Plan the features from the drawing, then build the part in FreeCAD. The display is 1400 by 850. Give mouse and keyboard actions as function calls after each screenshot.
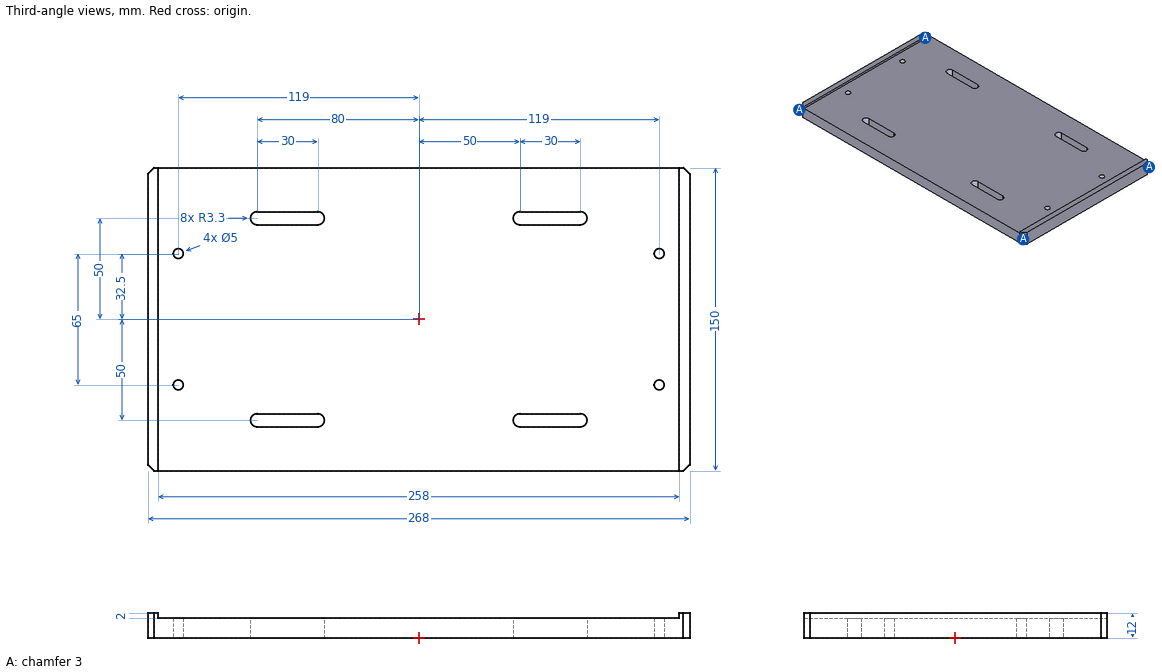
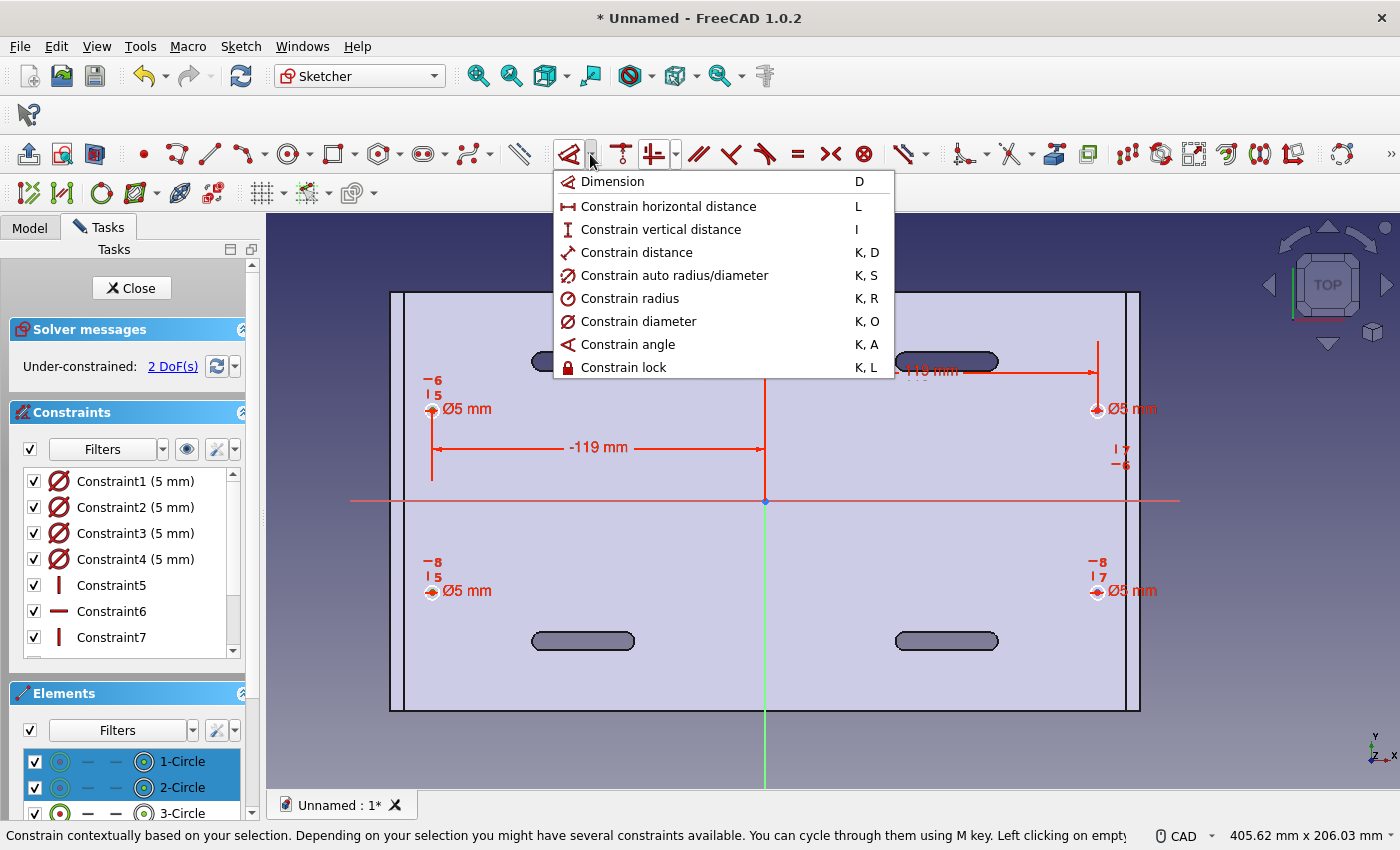
click(724, 230)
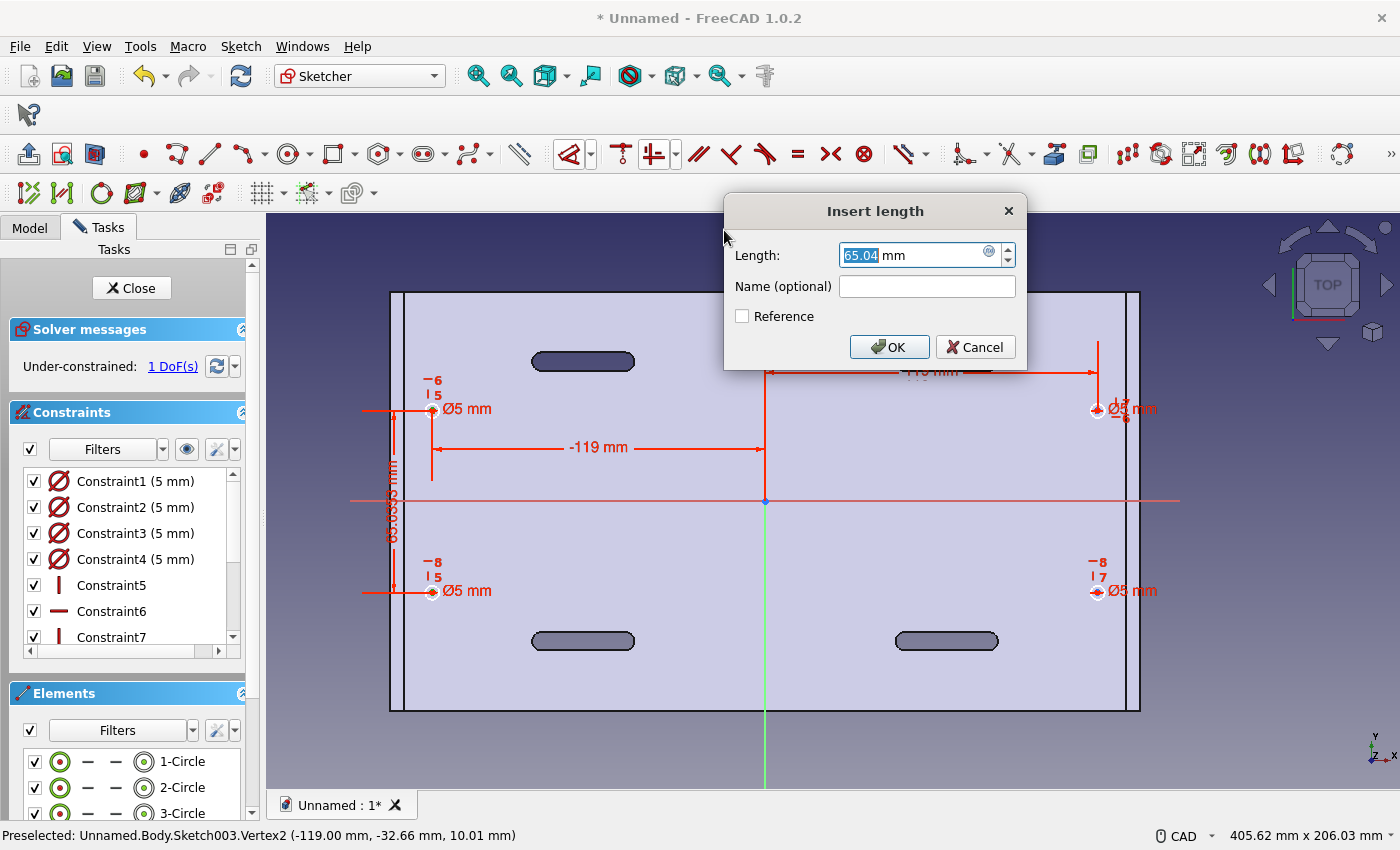
text(65)
key(Return)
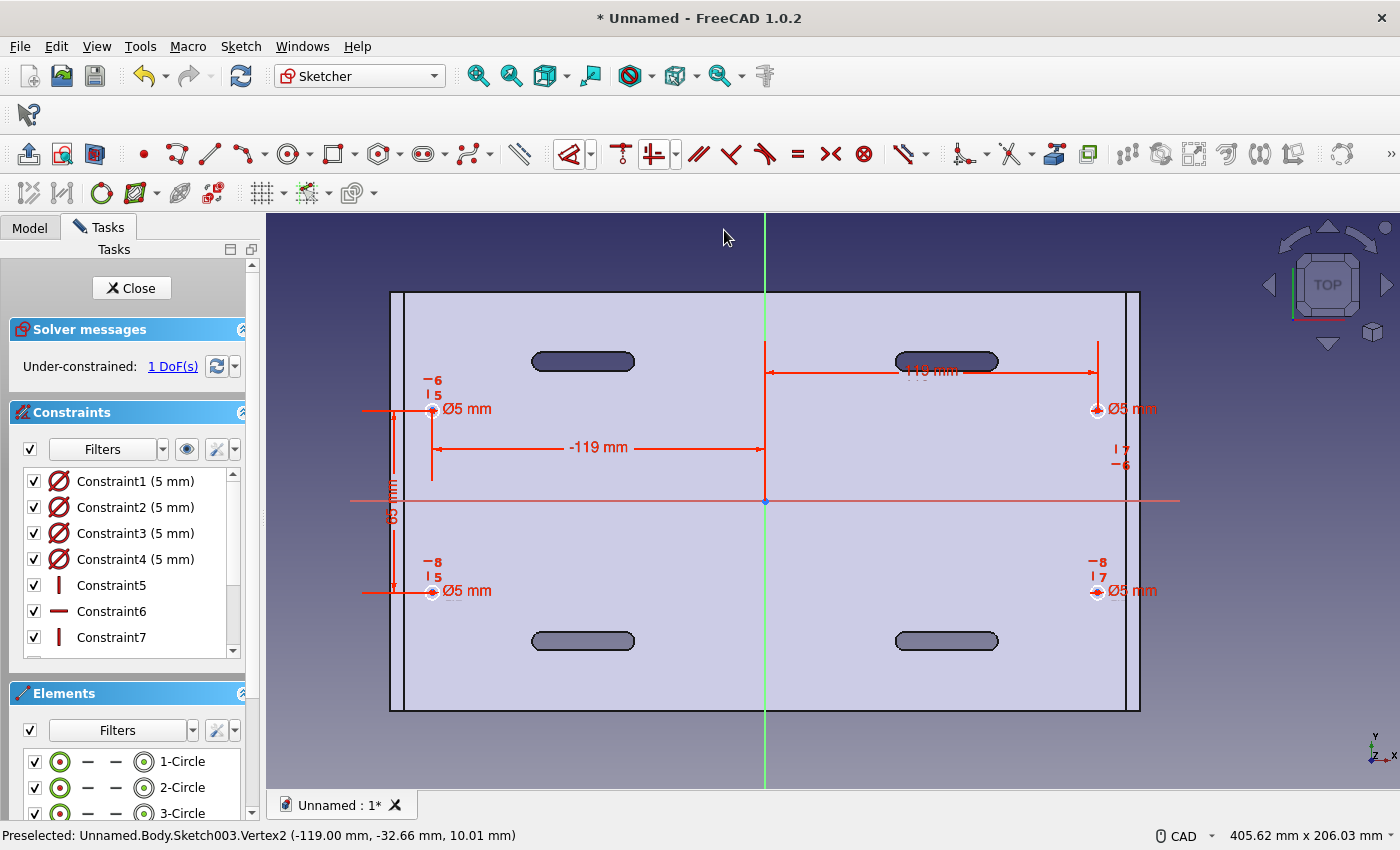
click(432, 411)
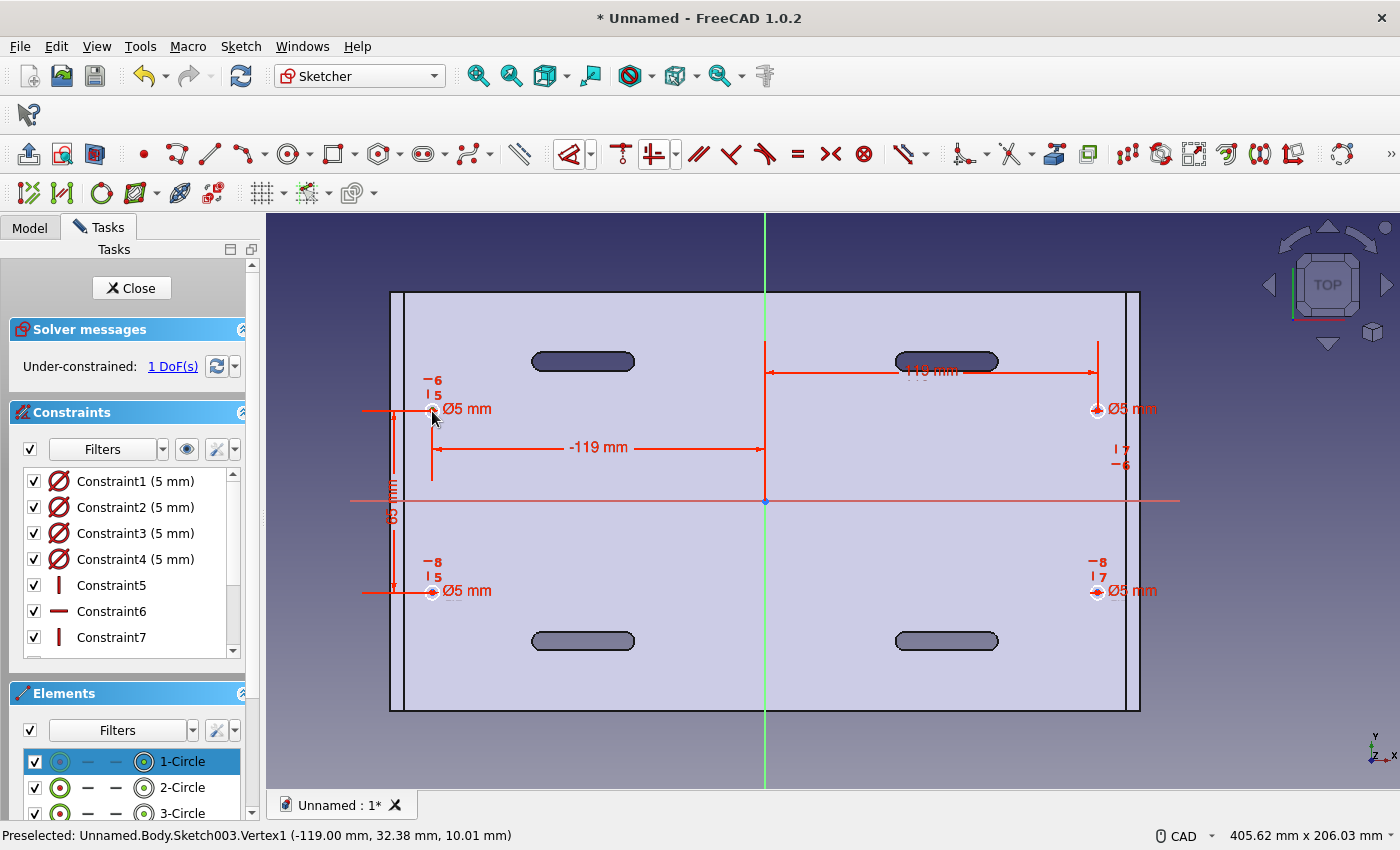
click(590, 154)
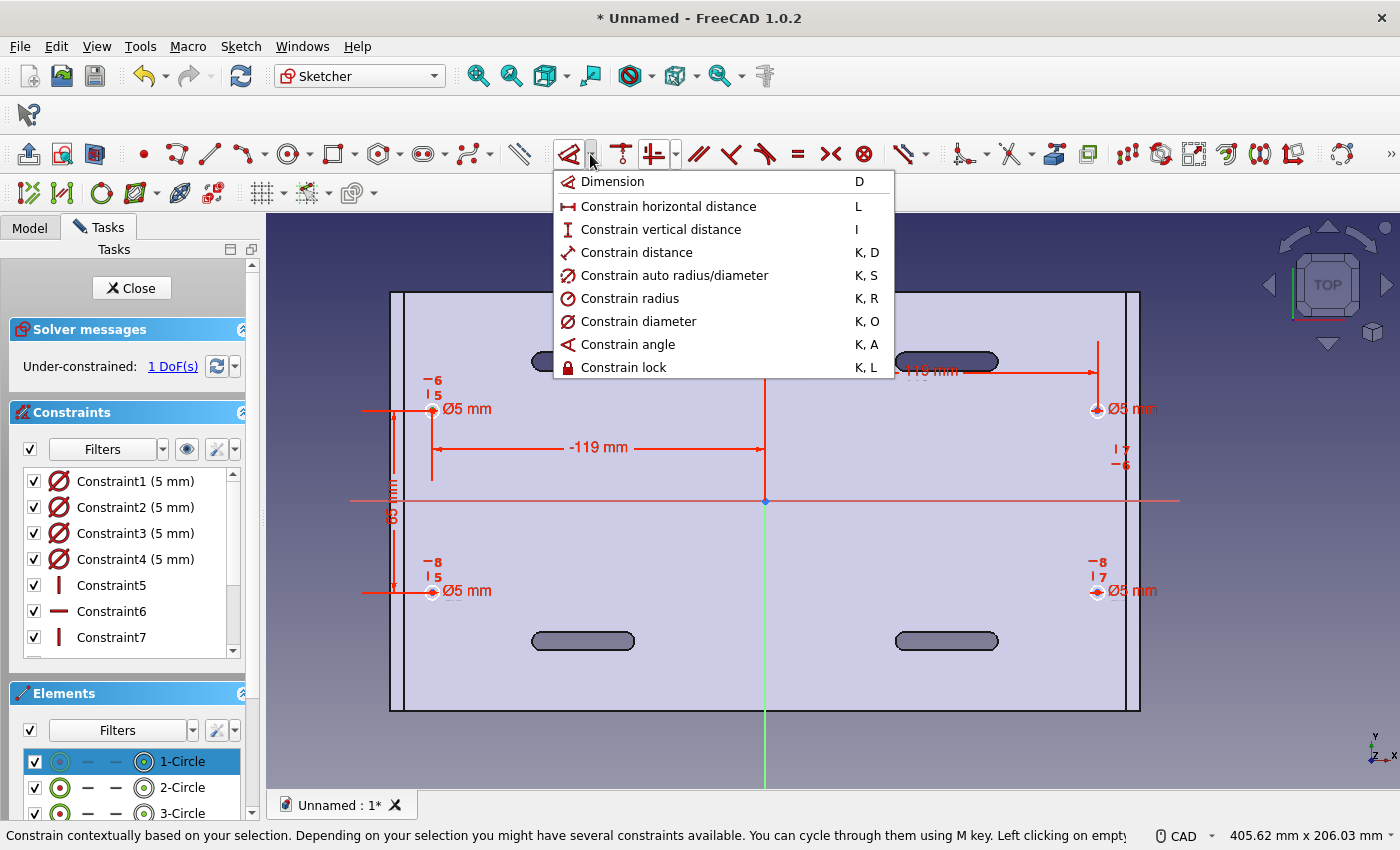
click(724, 230)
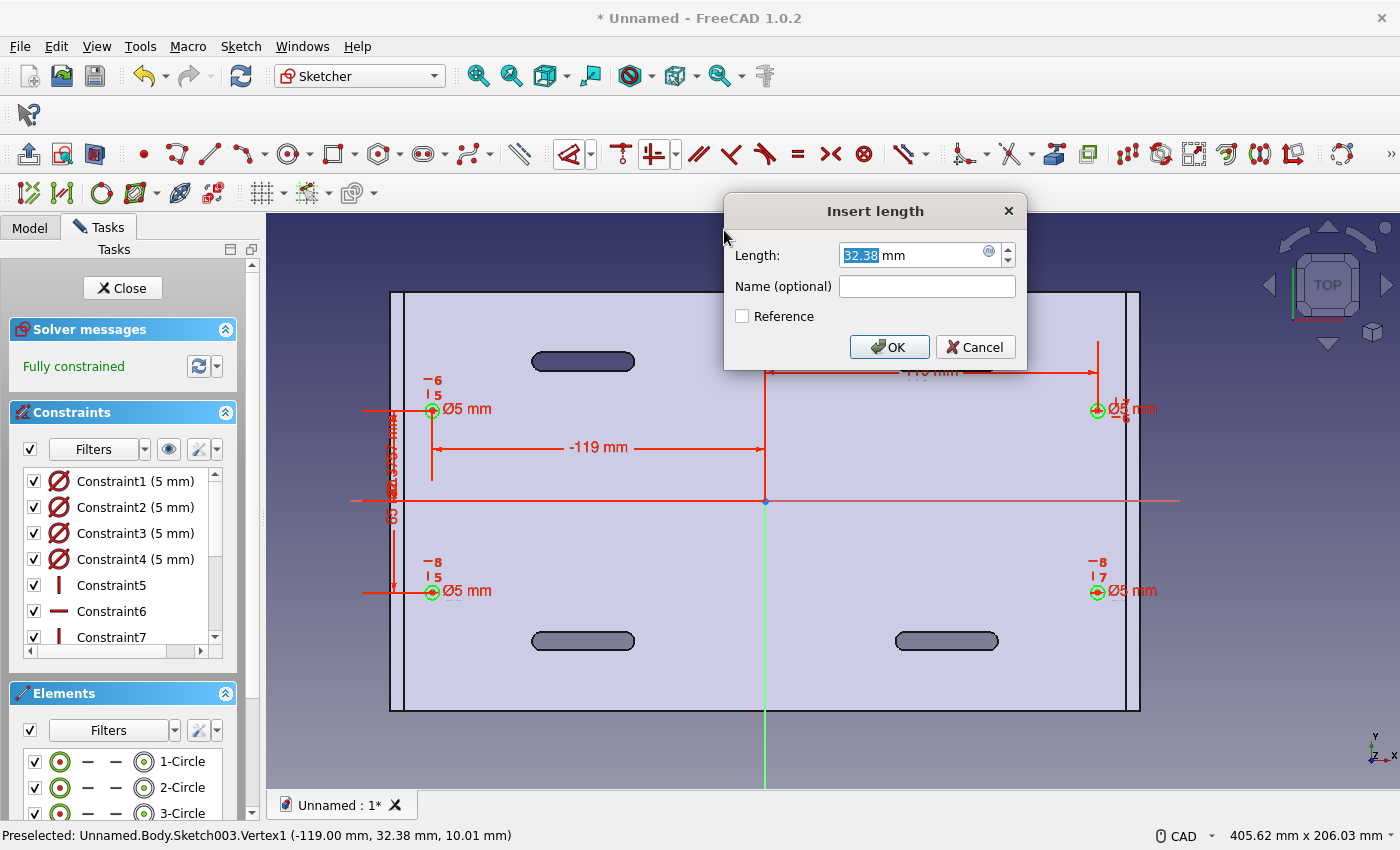
text(32.5)
key(Return)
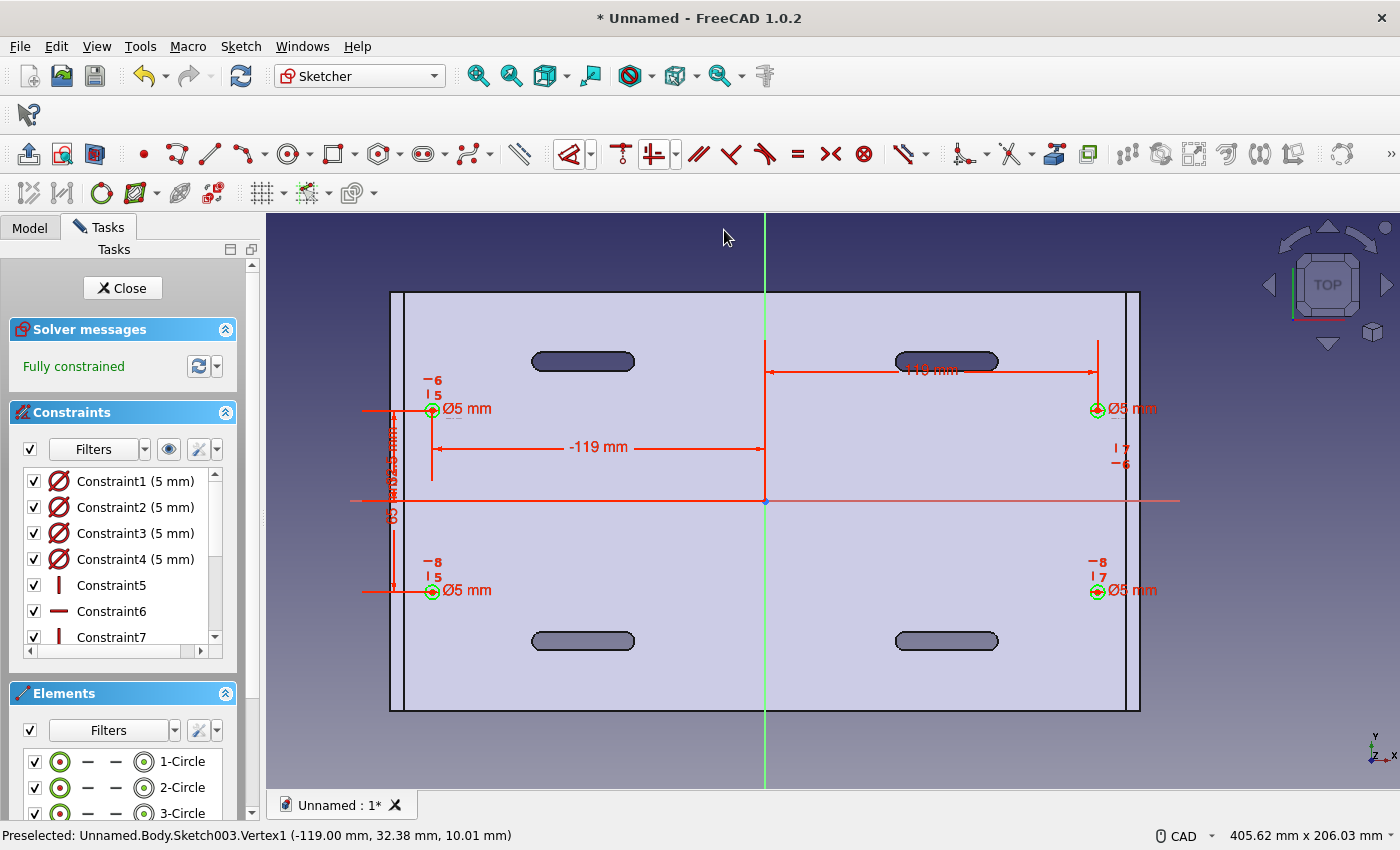
click(123, 288)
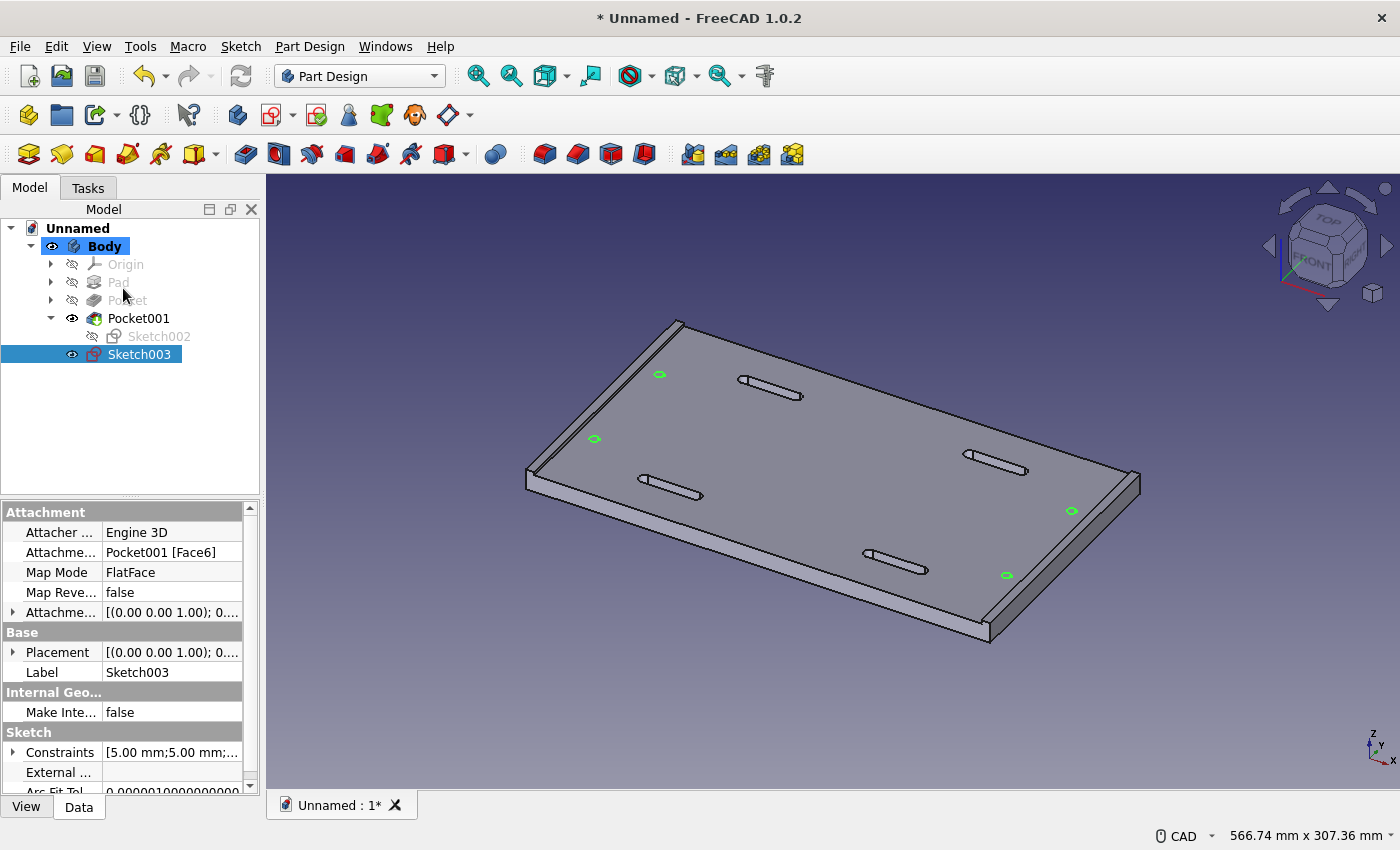
click(246, 154)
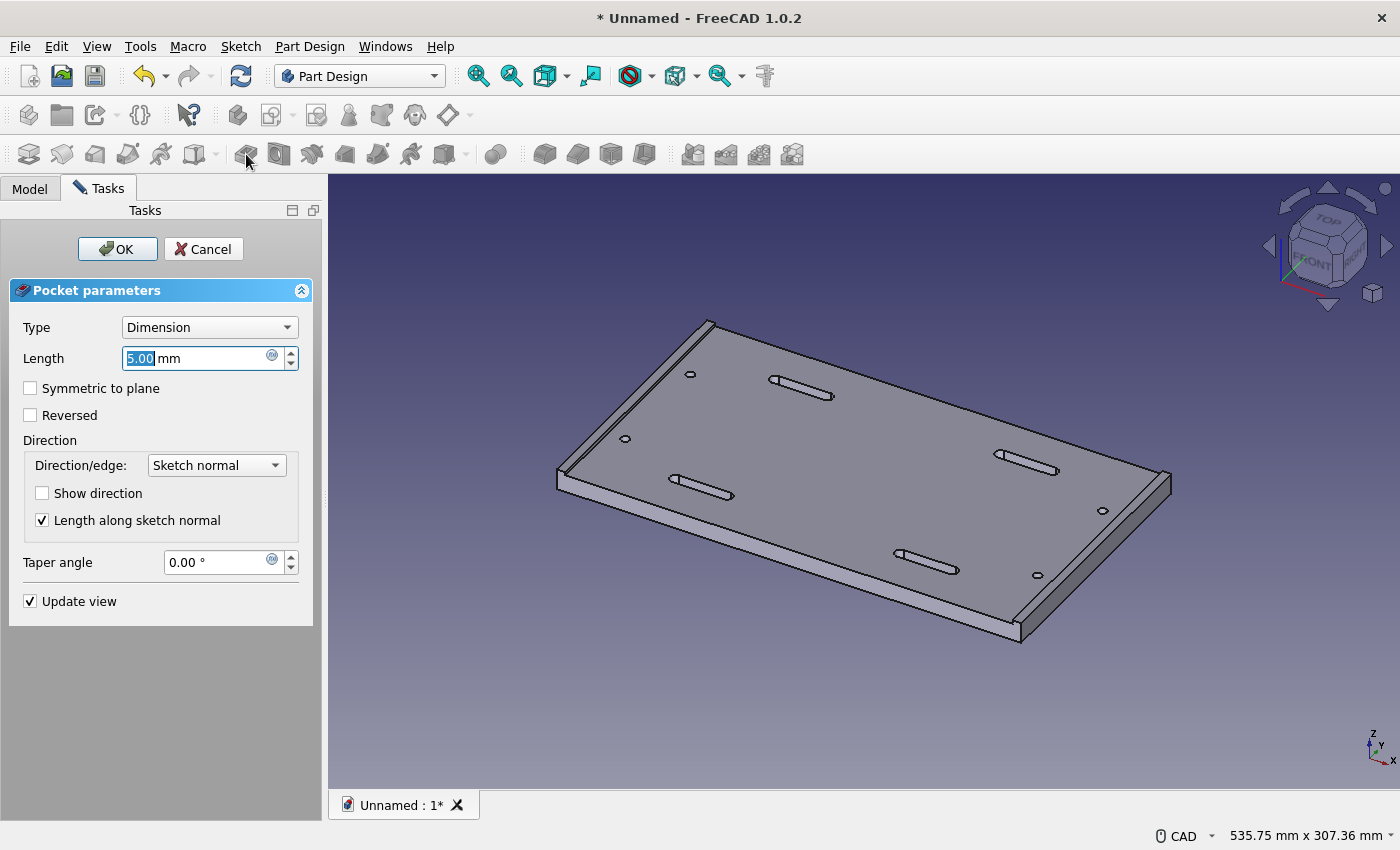
click(210, 328)